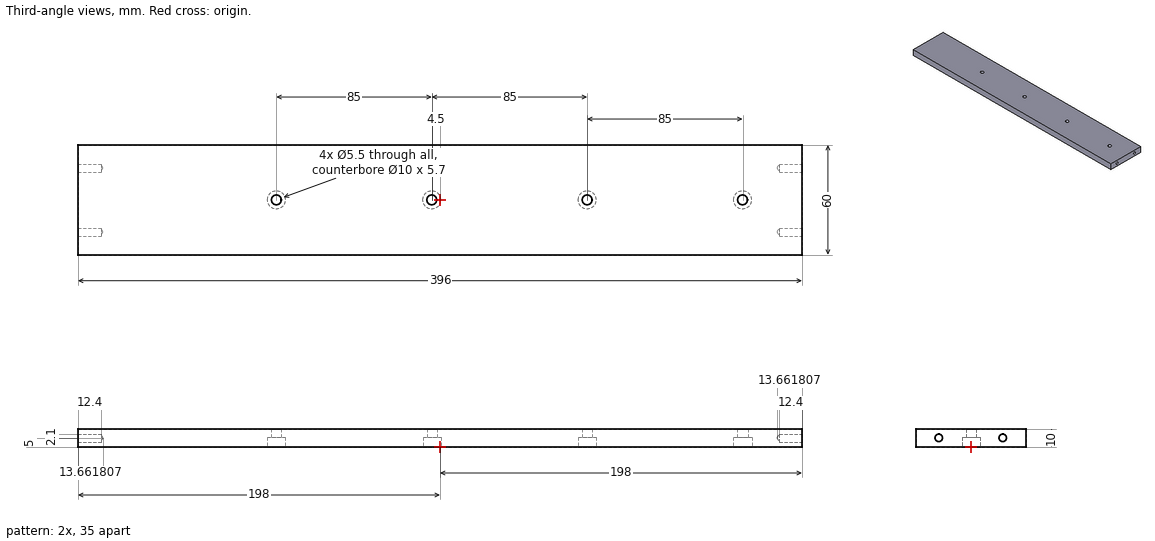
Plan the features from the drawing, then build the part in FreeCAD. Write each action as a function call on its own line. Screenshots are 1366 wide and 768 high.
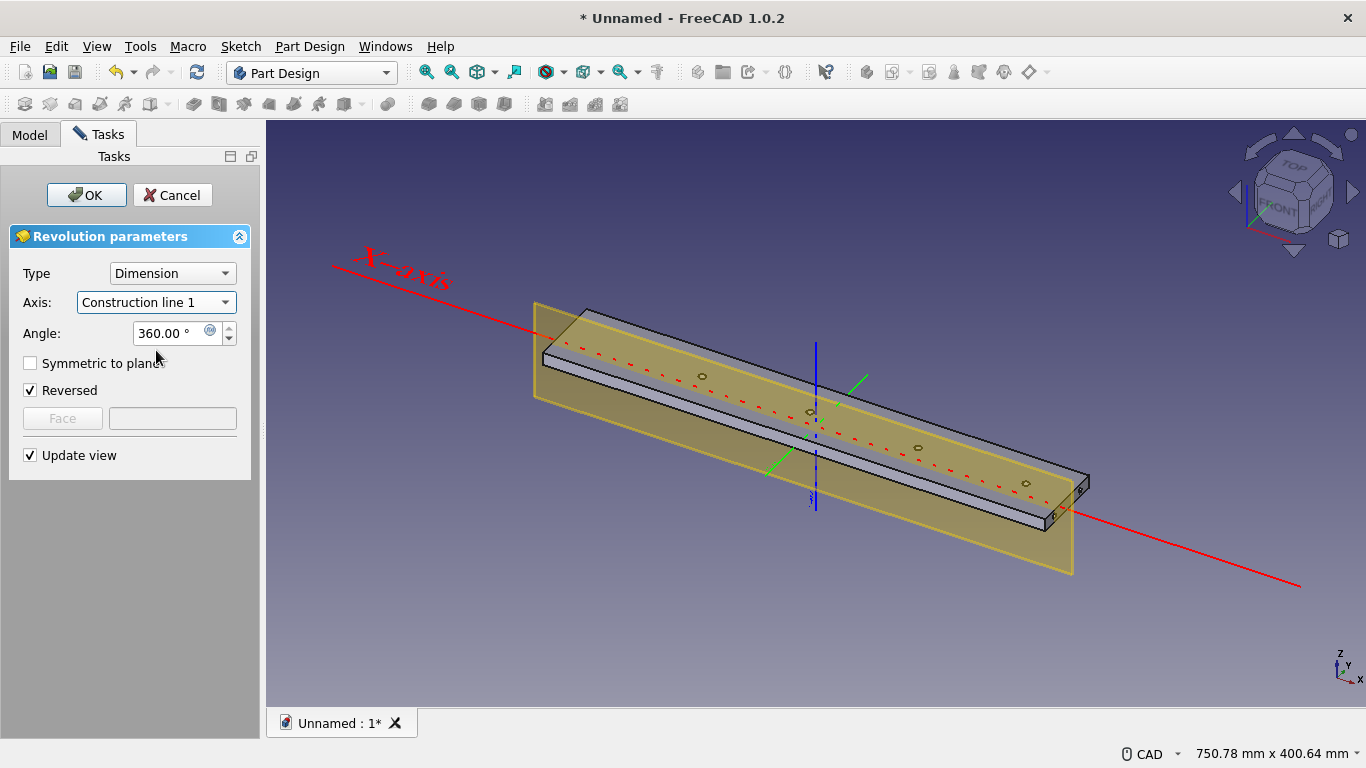
click(87, 195)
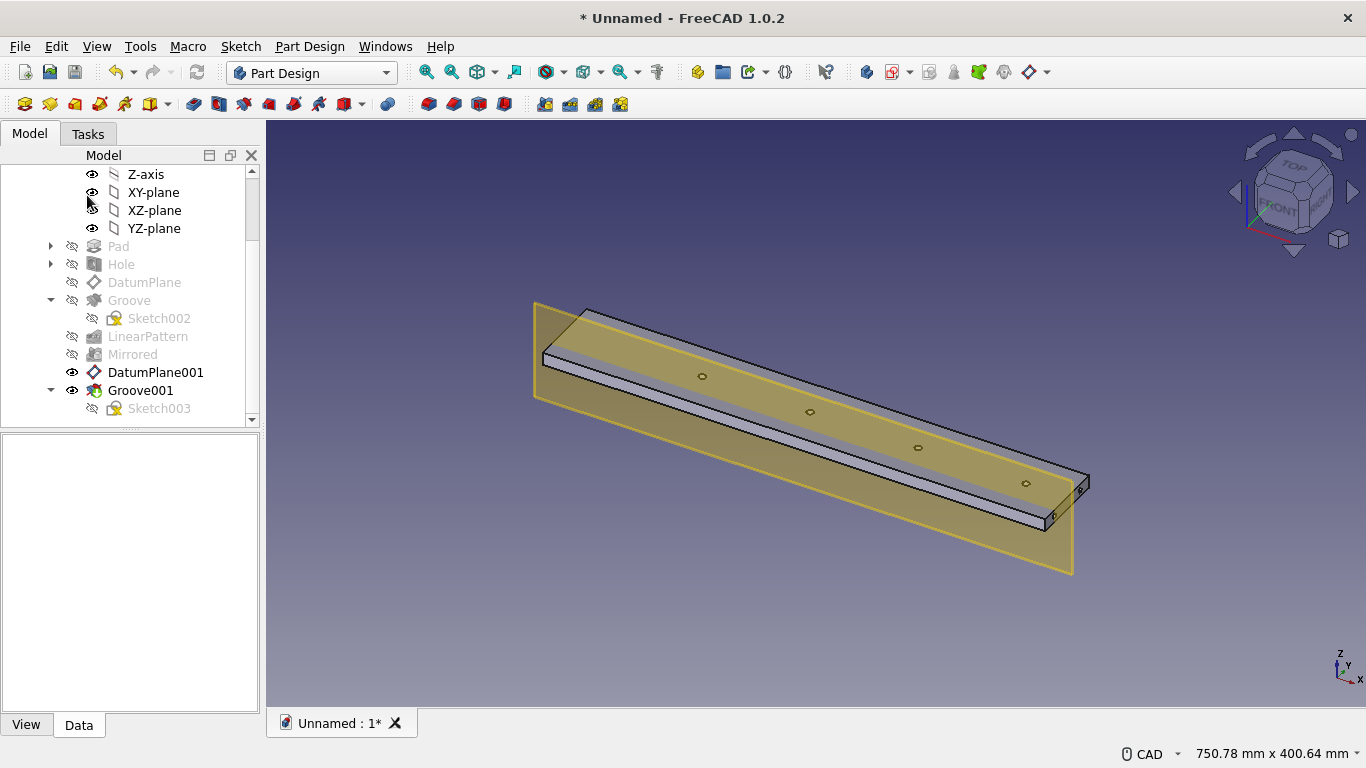
click(117, 372)
key(space)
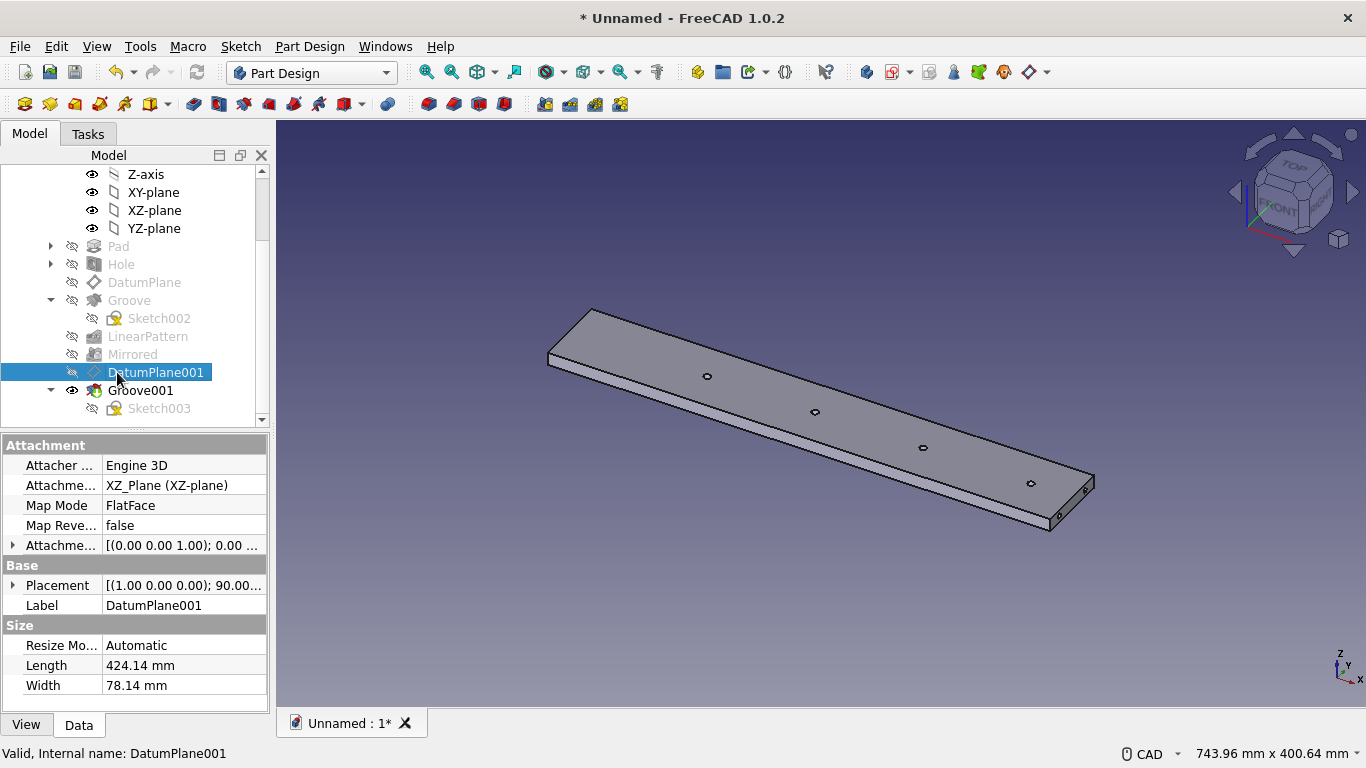
key(0)